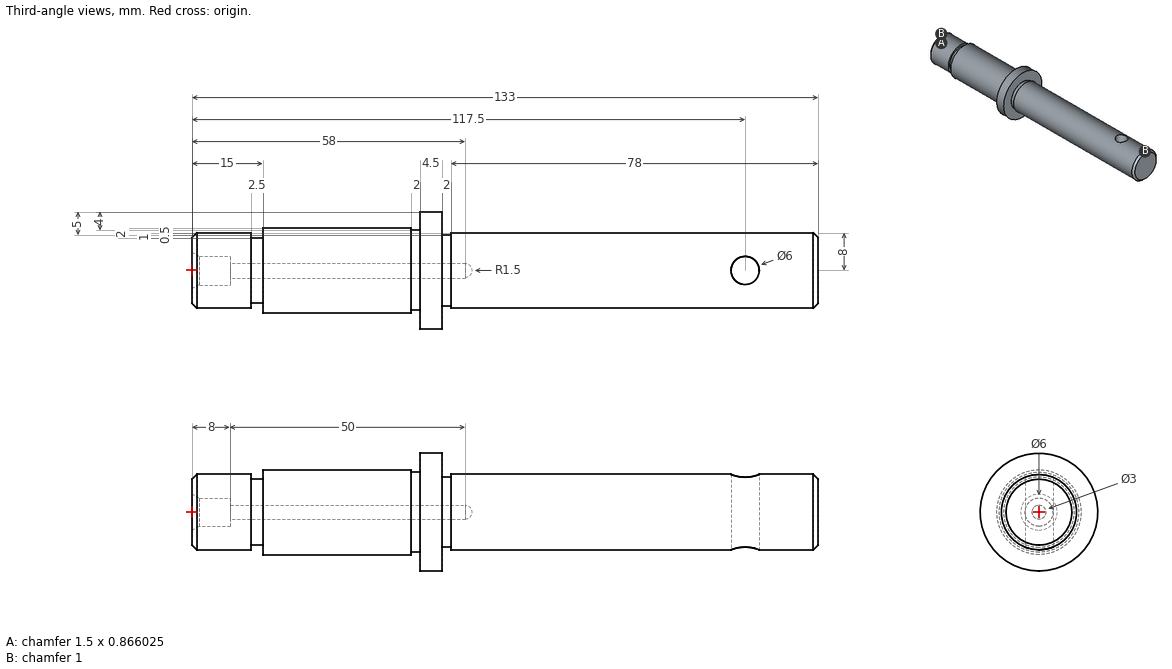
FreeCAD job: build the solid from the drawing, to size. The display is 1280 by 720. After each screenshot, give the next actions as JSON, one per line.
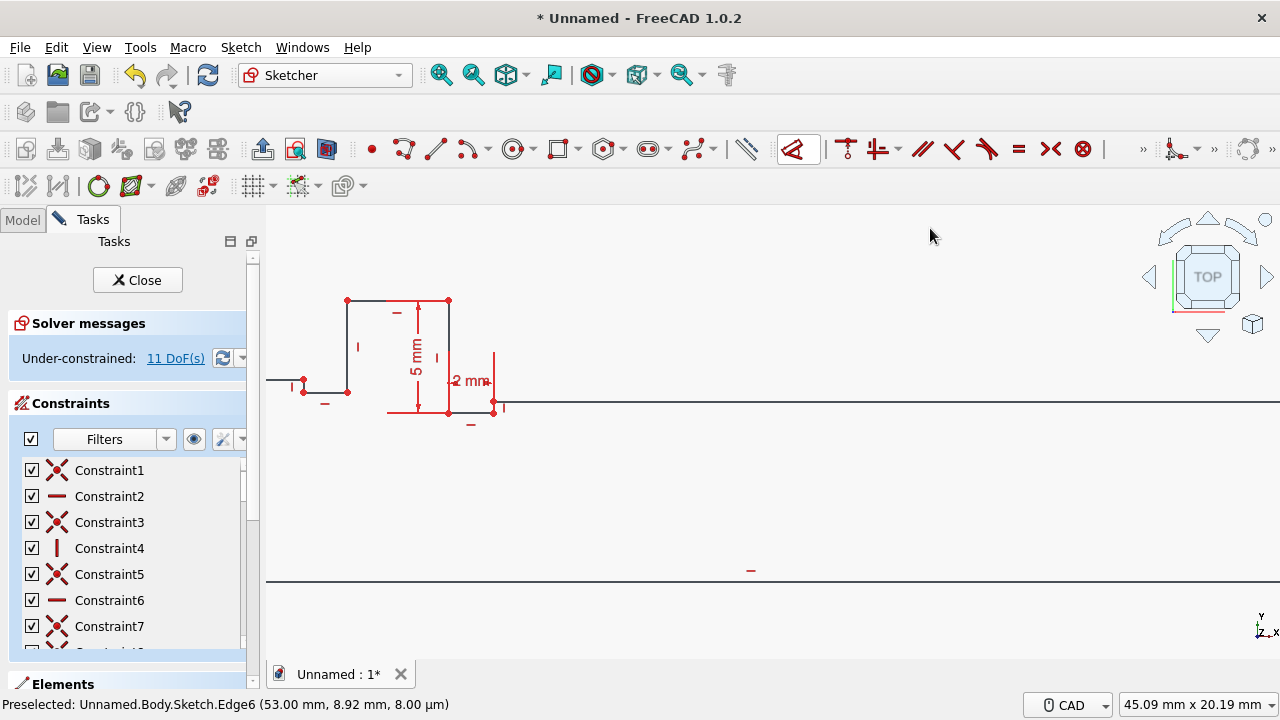
{"action": "left_click", "coordinate": [347, 328]}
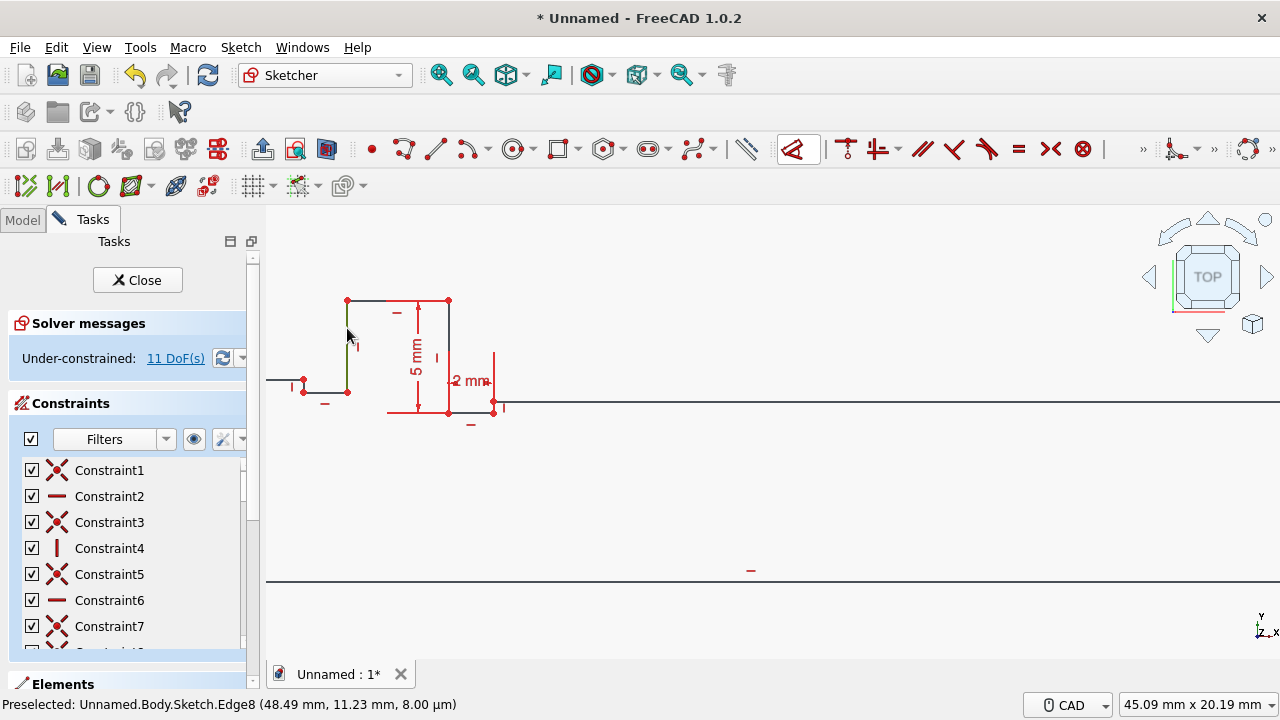
{"action": "key", "text": "i"}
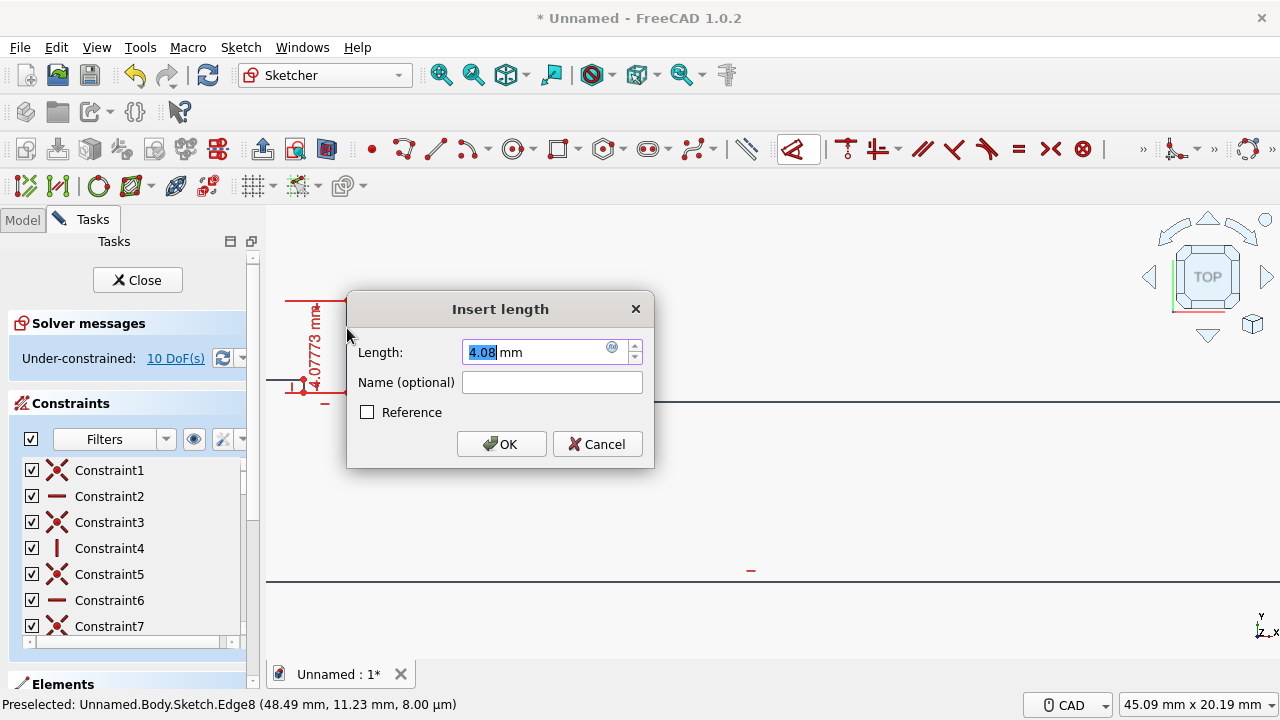
{"action": "type", "text": "4"}
{"action": "key", "text": "Return"}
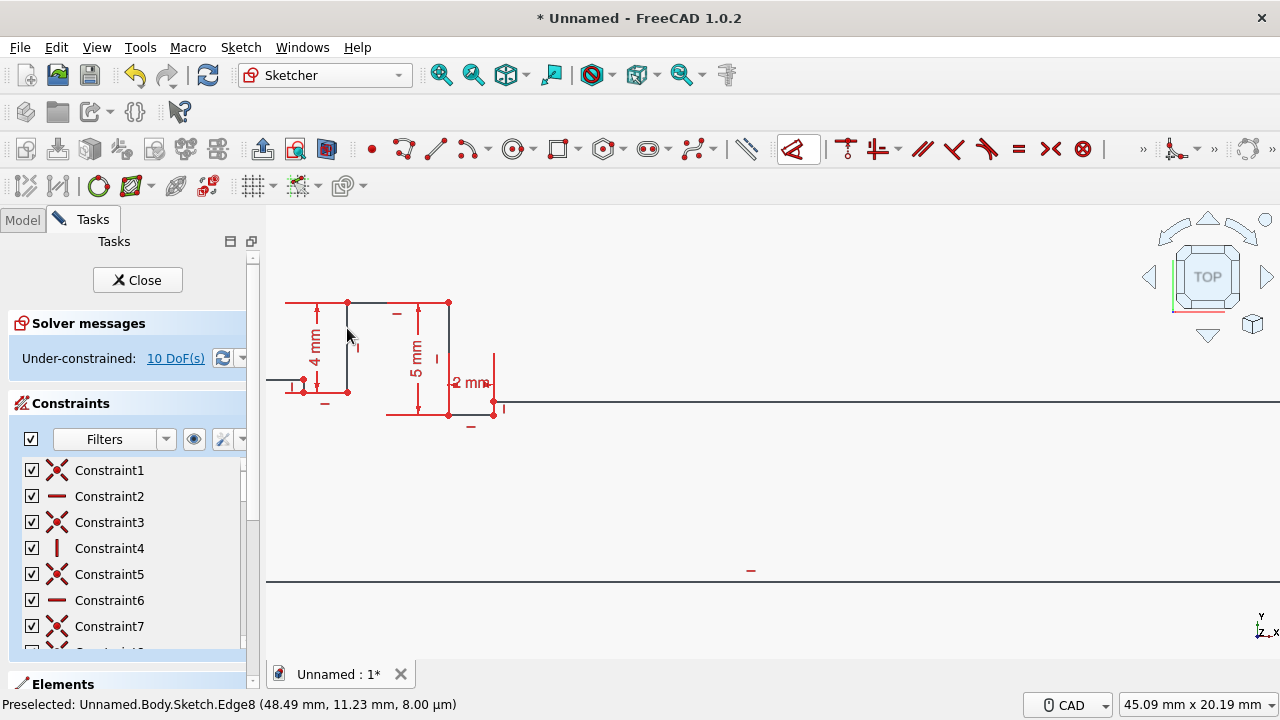
{"action": "left_click", "coordinate": [334, 393]}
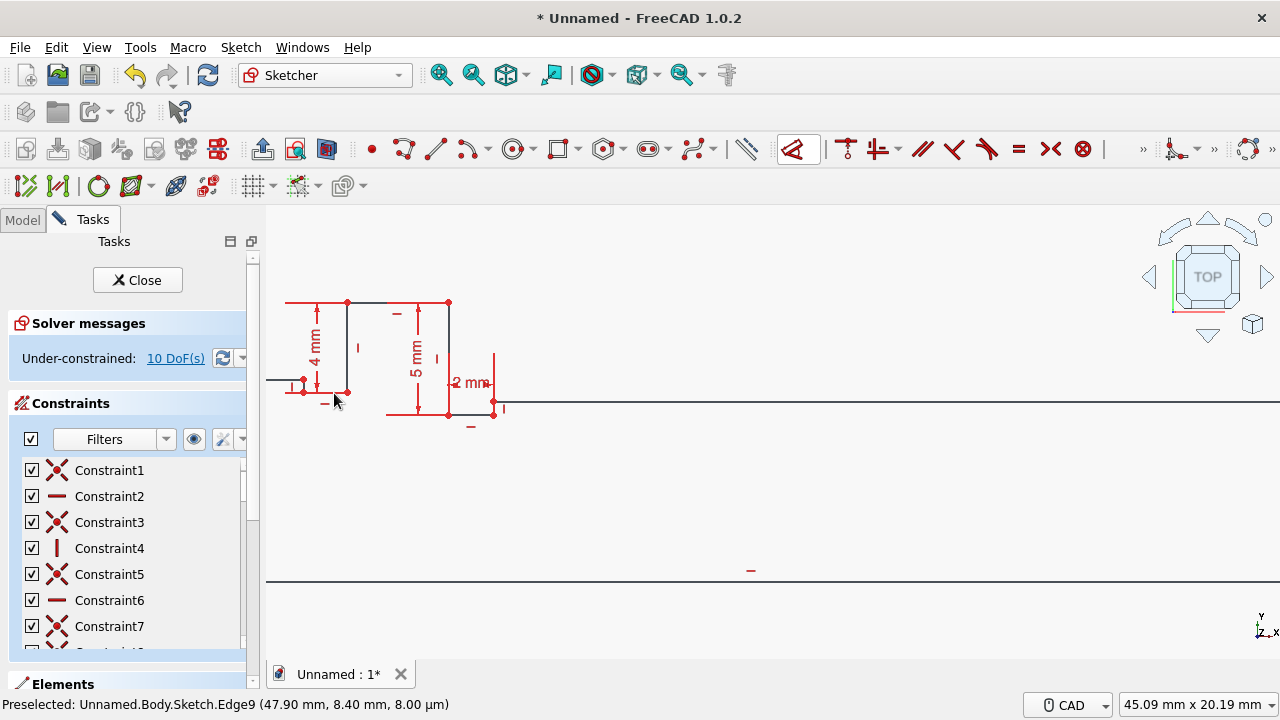
{"action": "key", "text": "l"}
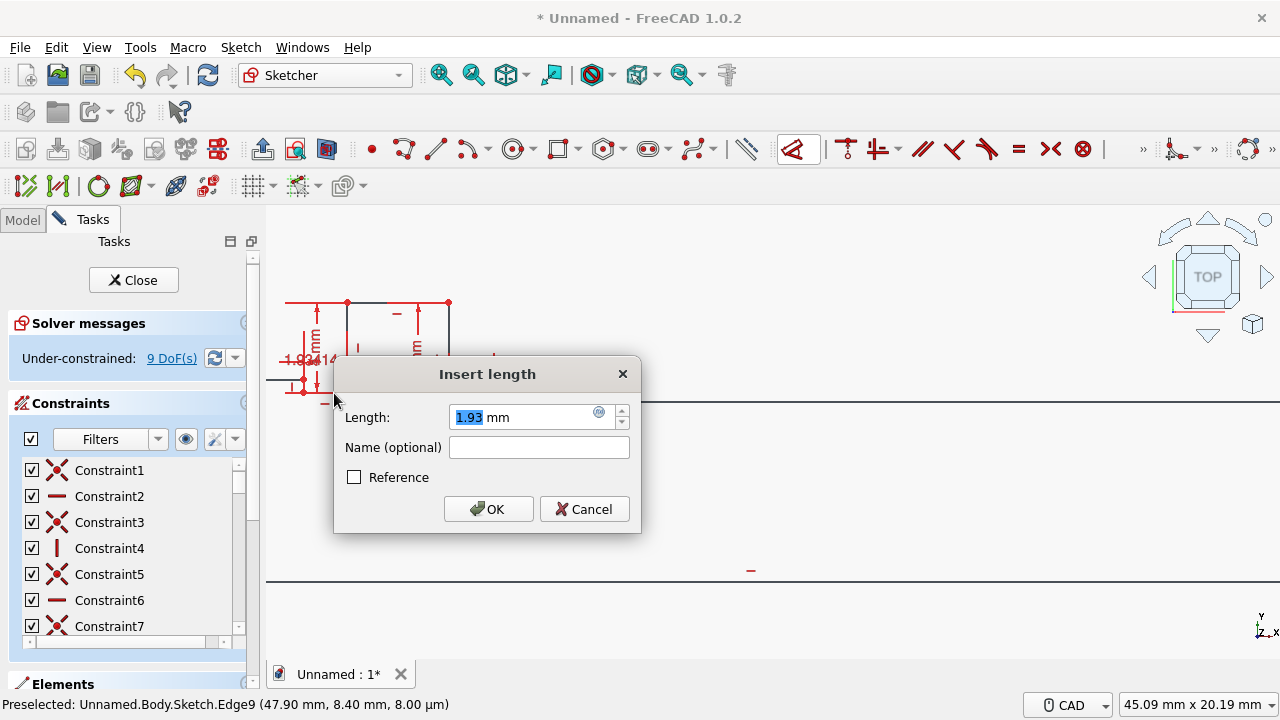
{"action": "type", "text": "2"}
{"action": "key", "text": "Return"}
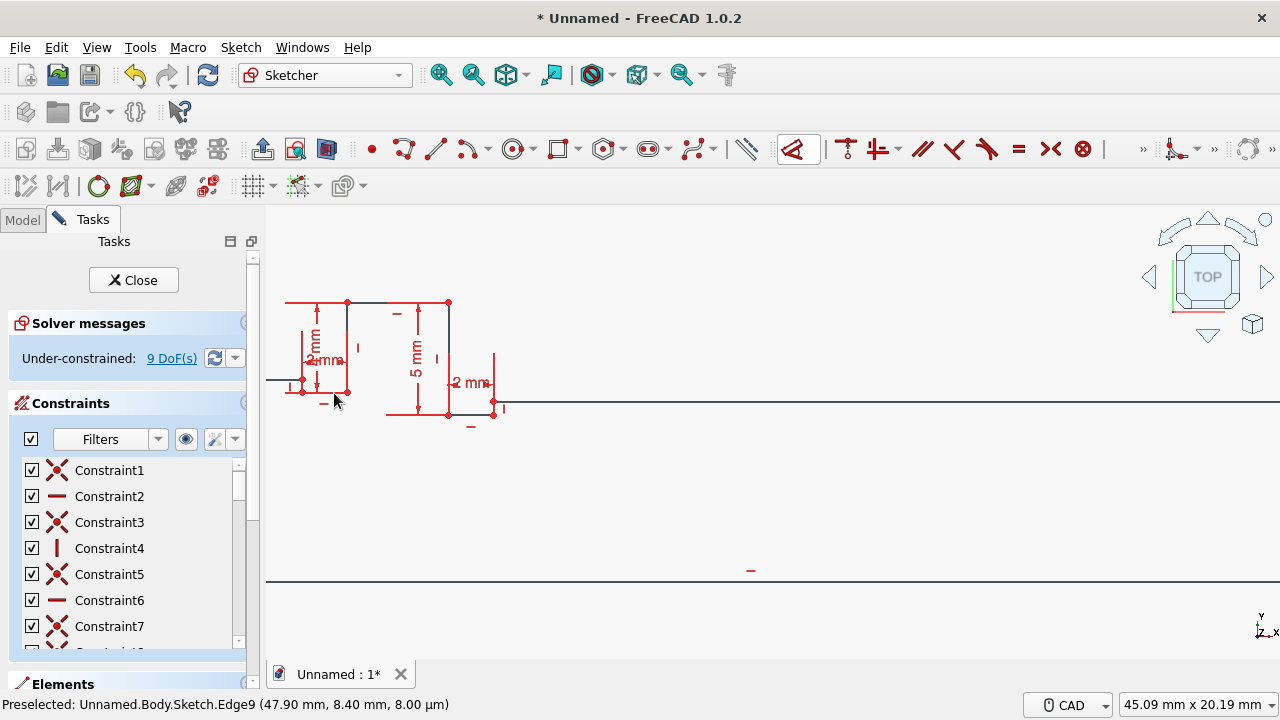
{"action": "scroll", "coordinate": [692, 430], "scroll_direction": "down", "scroll_amount": 8}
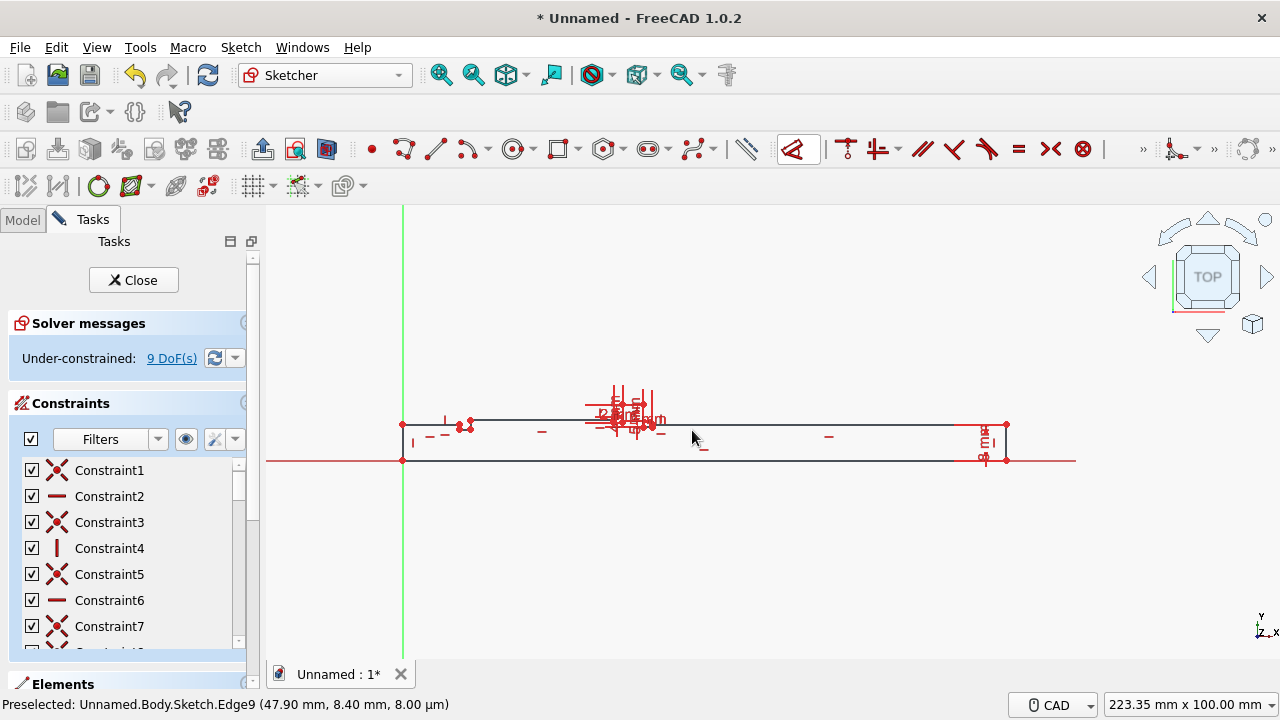
{"action": "scroll", "coordinate": [471, 423], "scroll_direction": "up", "scroll_amount": 8}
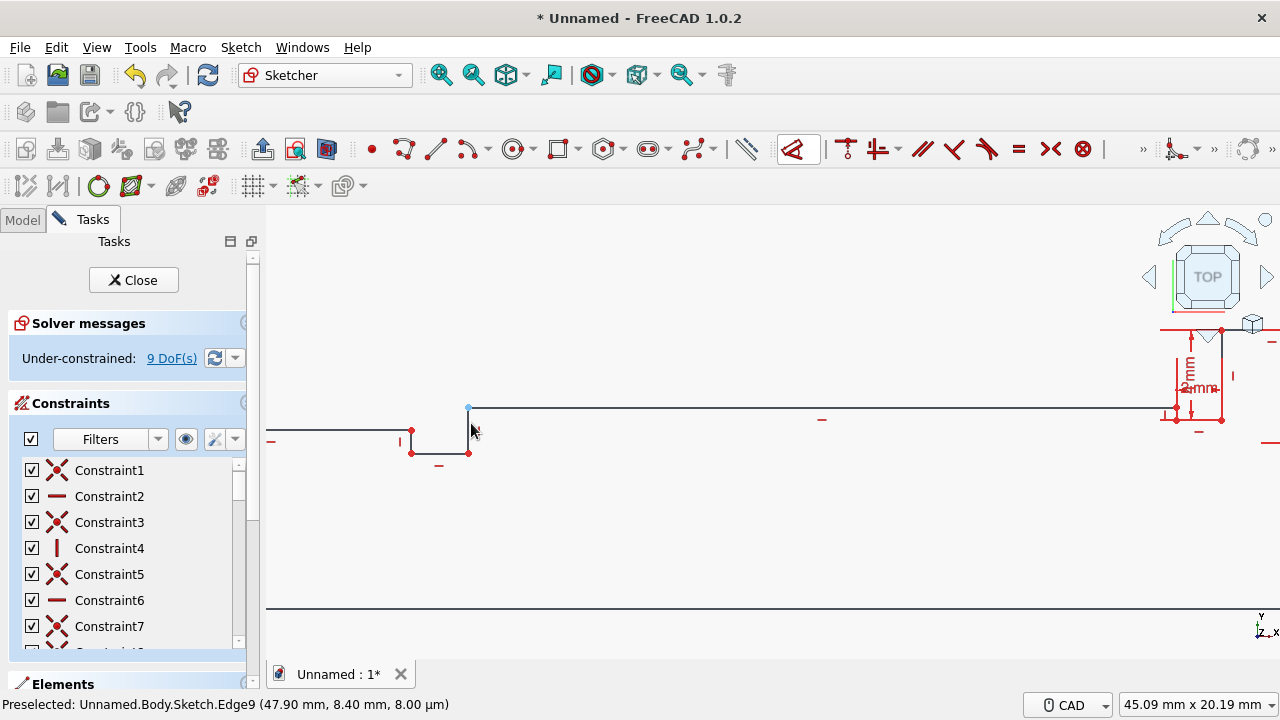
{"action": "left_click", "coordinate": [468, 422]}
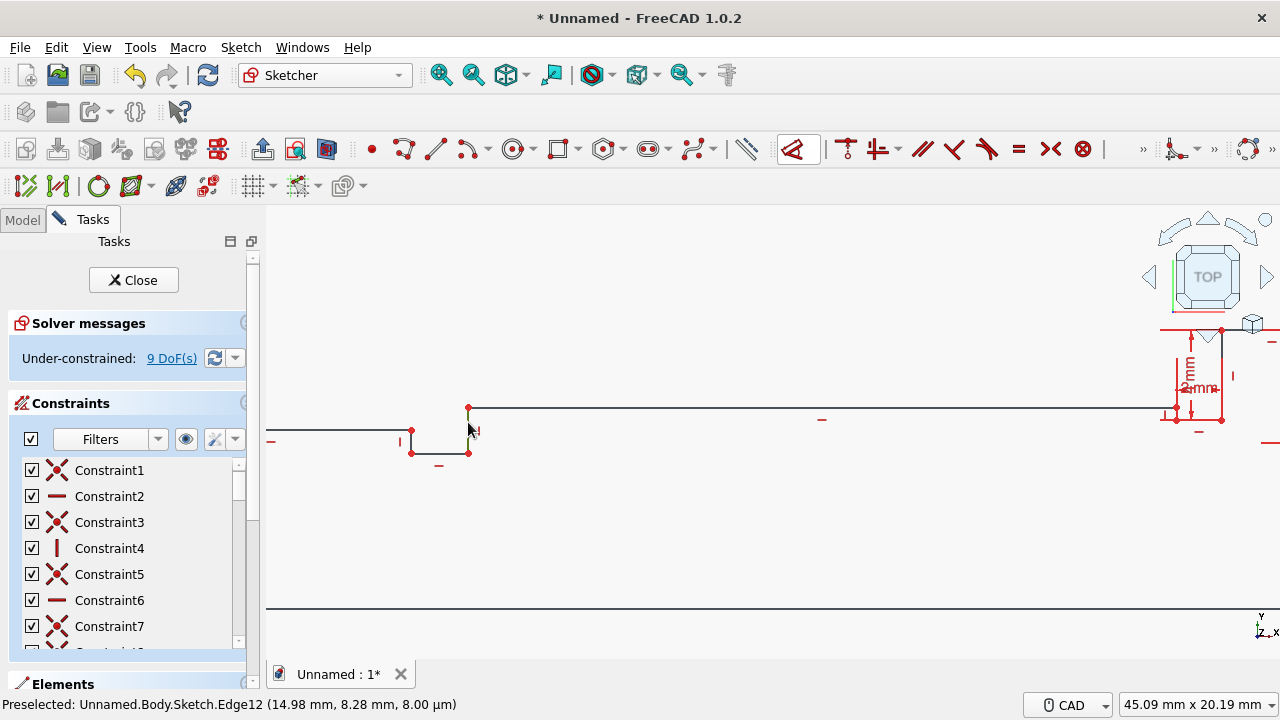
{"action": "key", "text": "i"}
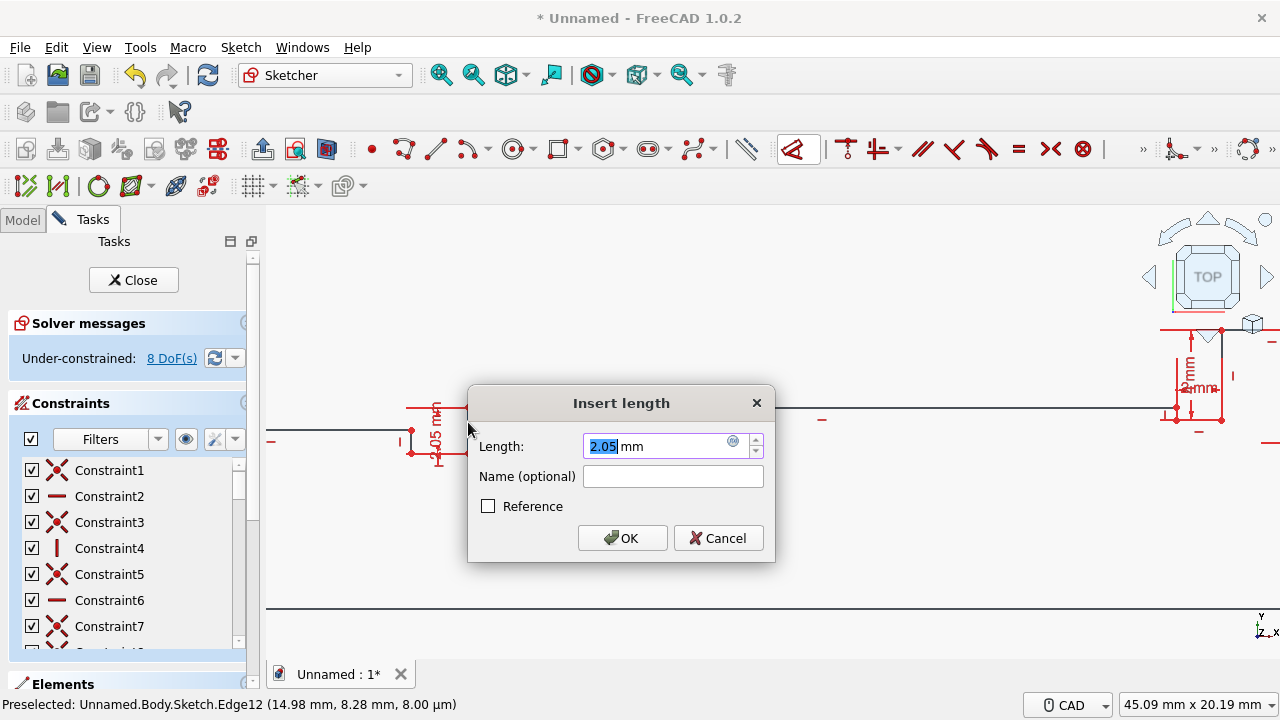
{"action": "type", "text": "2"}
{"action": "key", "text": "Return"}